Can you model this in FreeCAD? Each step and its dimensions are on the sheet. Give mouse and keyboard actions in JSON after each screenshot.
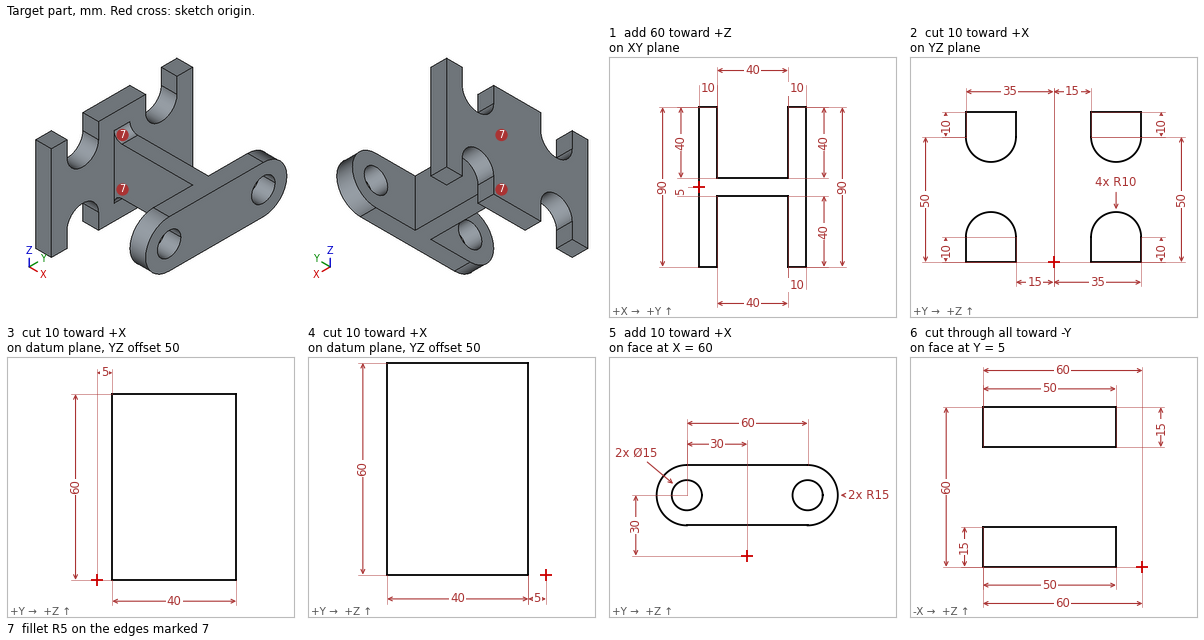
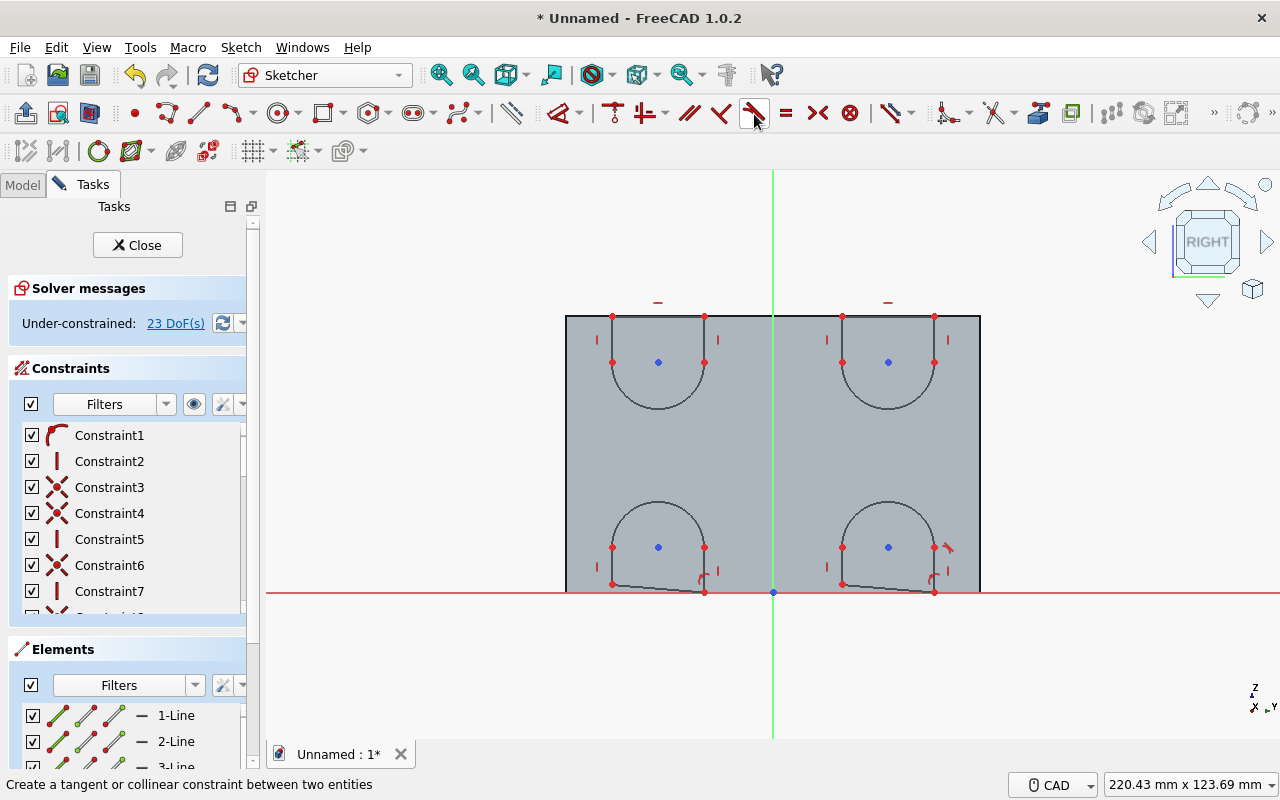
{"action": "scroll", "coordinate": [842, 574], "scroll_direction": "up", "scroll_amount": 2}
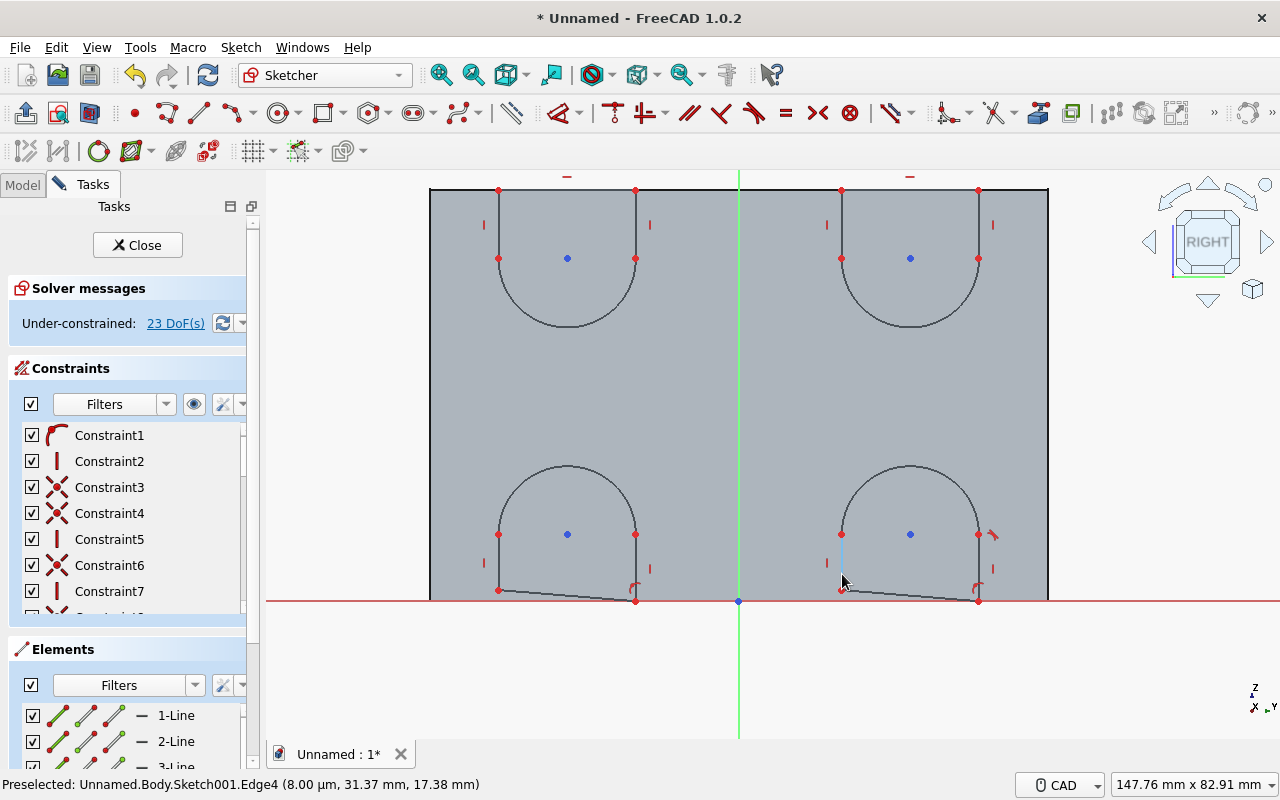
{"action": "left_click", "coordinate": [842, 574]}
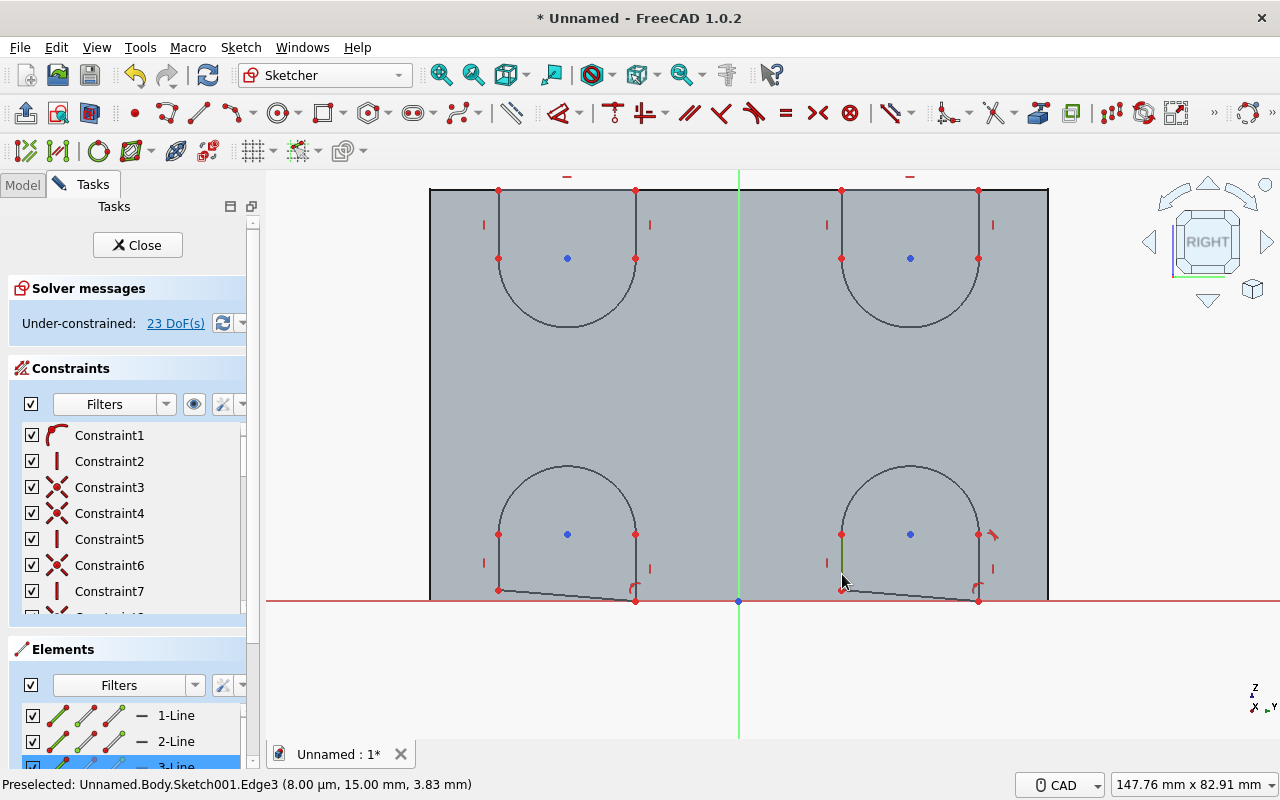
{"action": "left_click", "coordinate": [951, 479]}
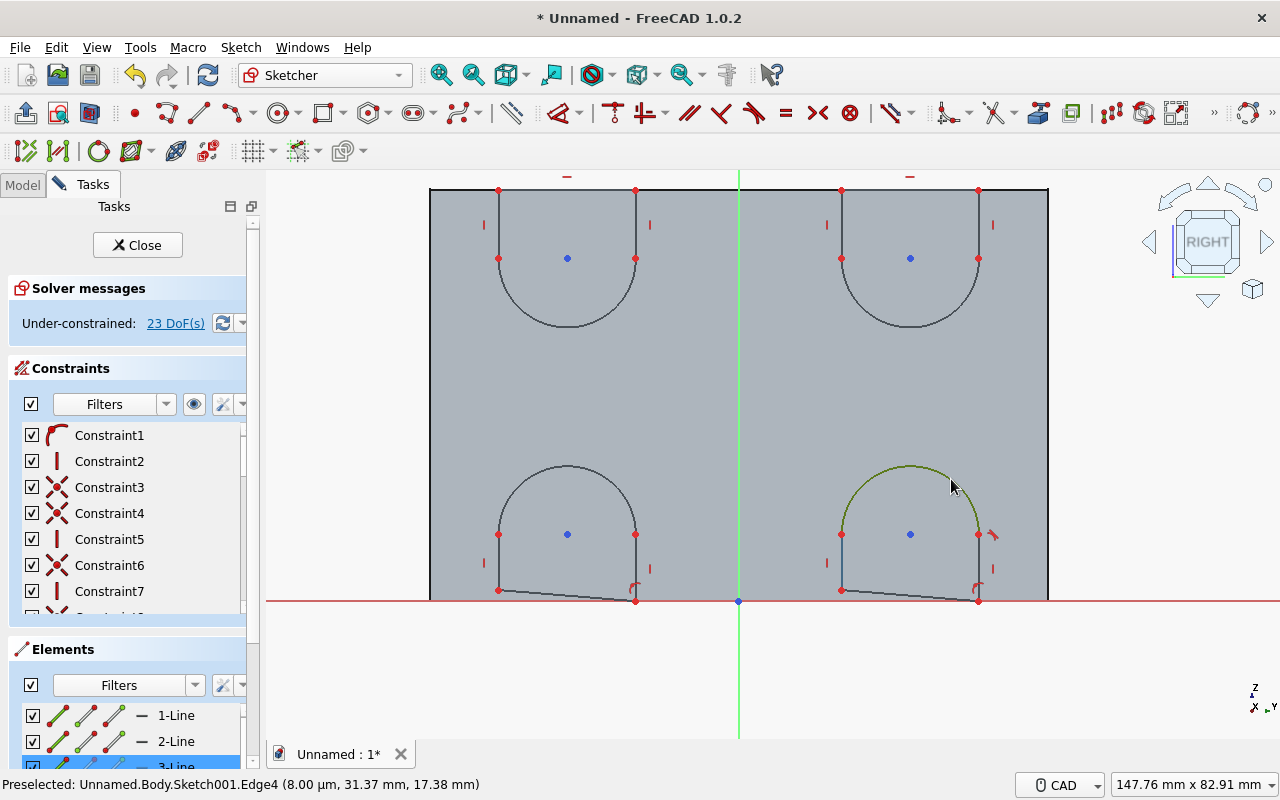
{"action": "left_click", "coordinate": [754, 114]}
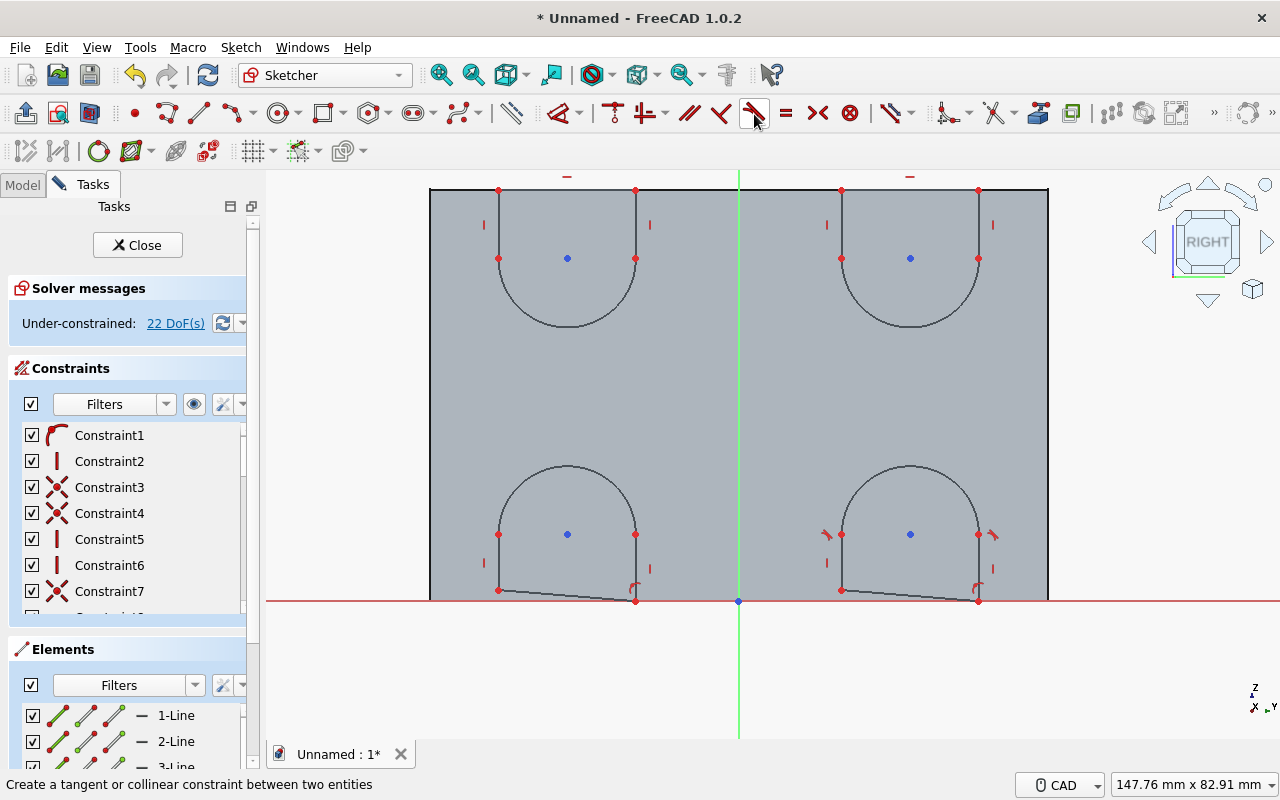
{"action": "left_click", "coordinate": [842, 238]}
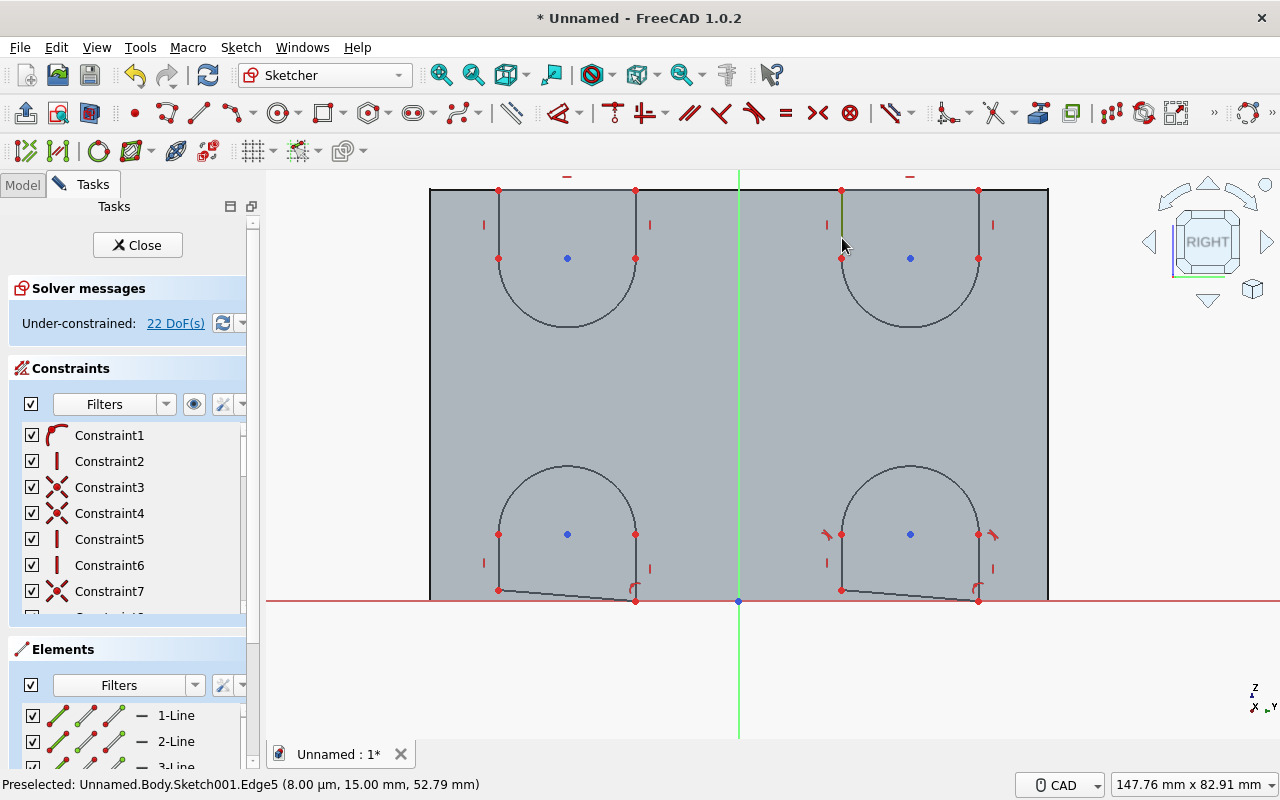
{"action": "left_click", "coordinate": [870, 314]}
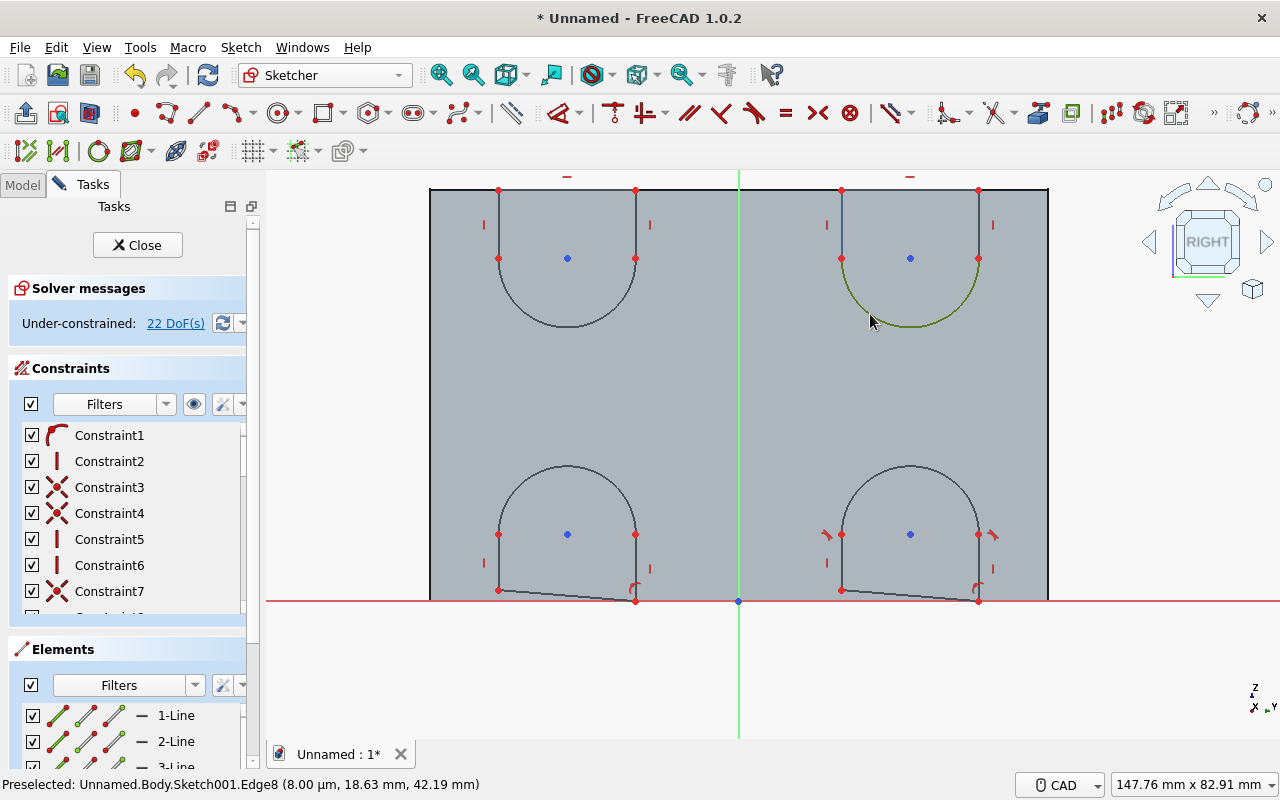
{"action": "left_click", "coordinate": [754, 114]}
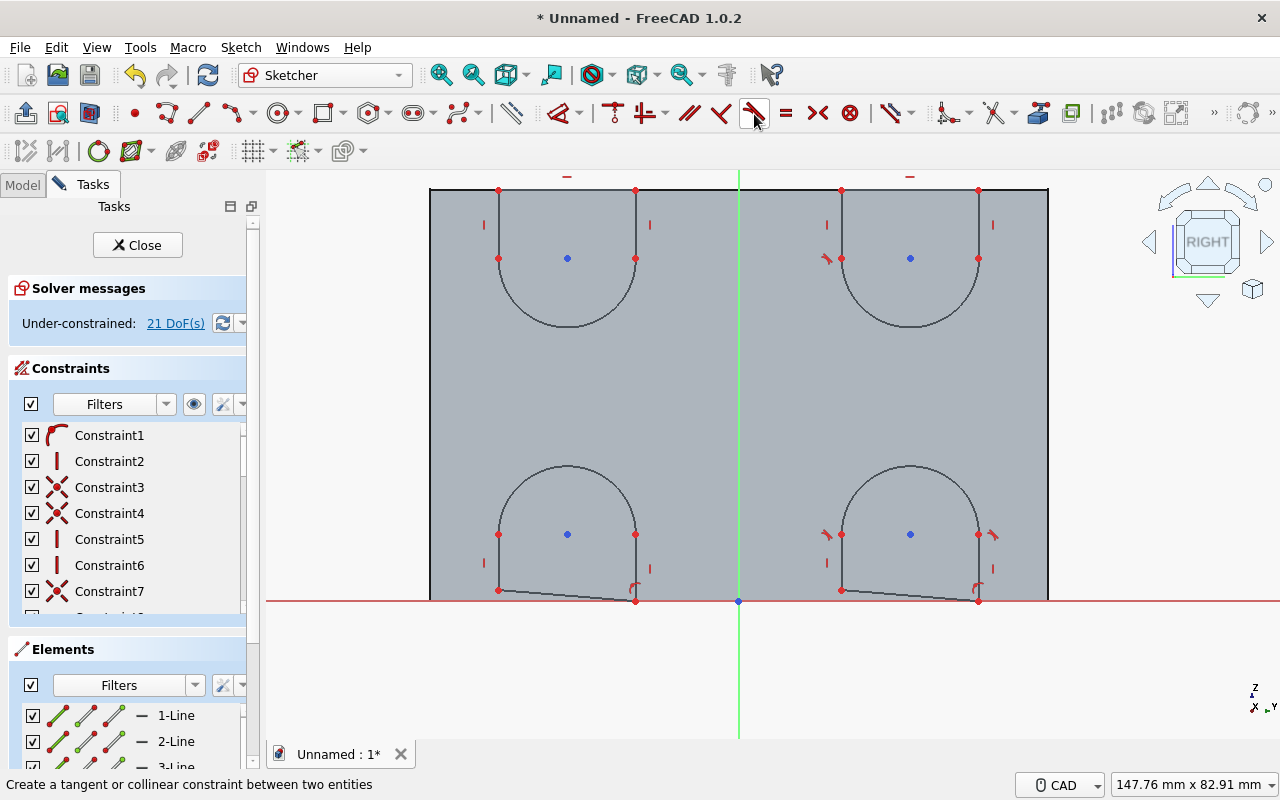
{"action": "left_click", "coordinate": [979, 211]}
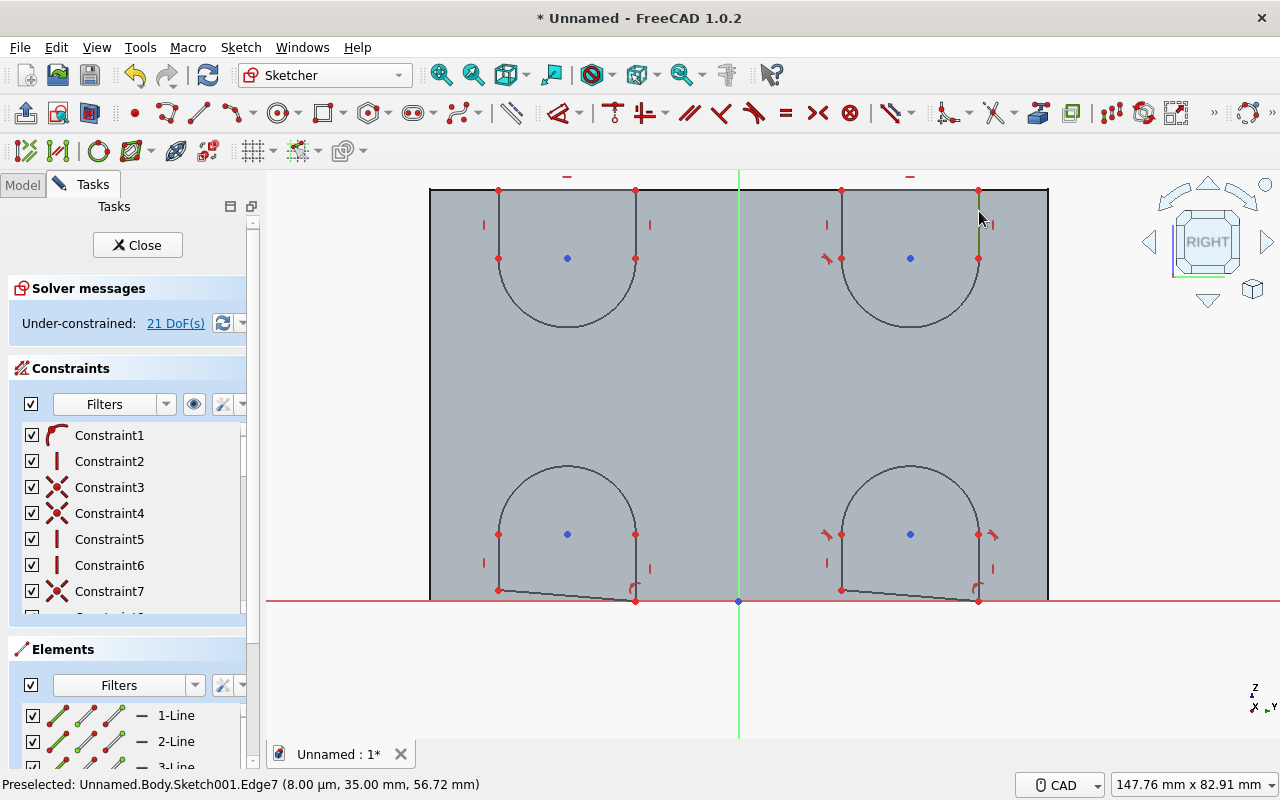
{"action": "left_click", "coordinate": [870, 314]}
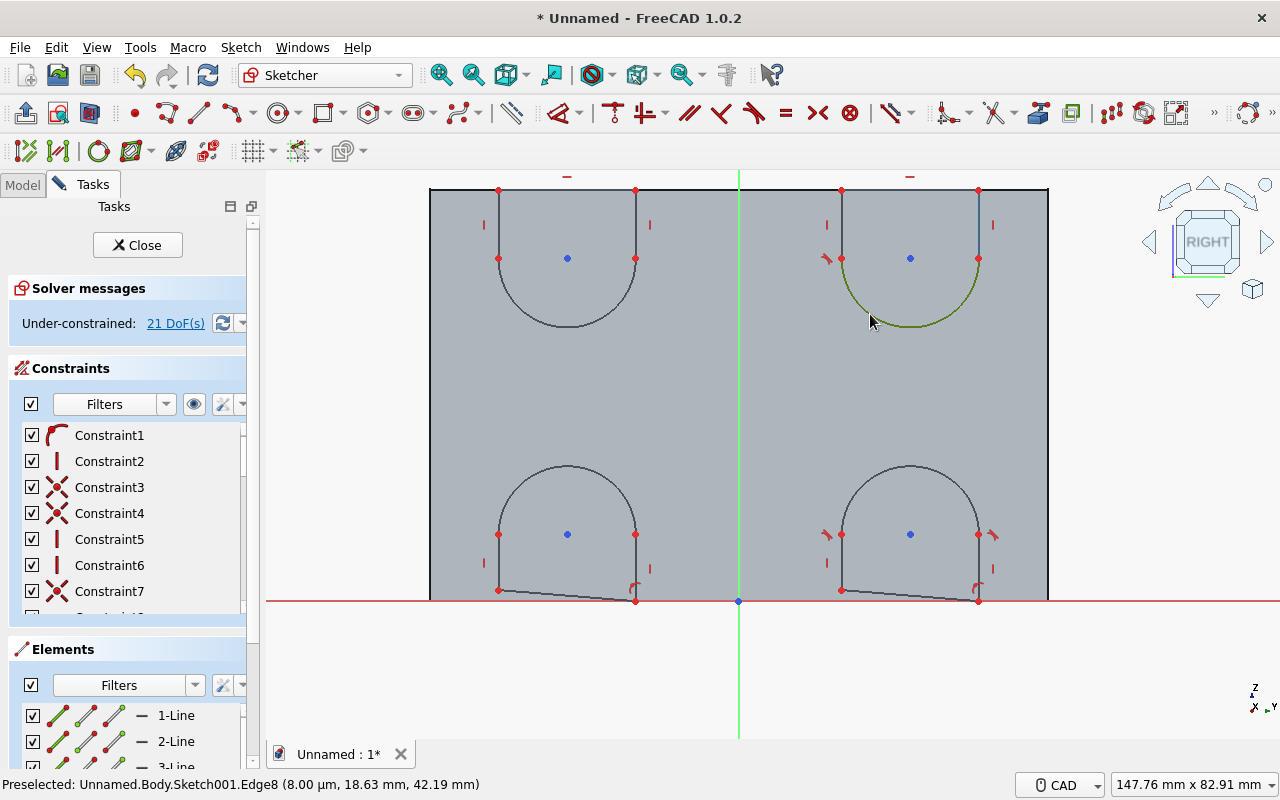
{"action": "left_click", "coordinate": [754, 114]}